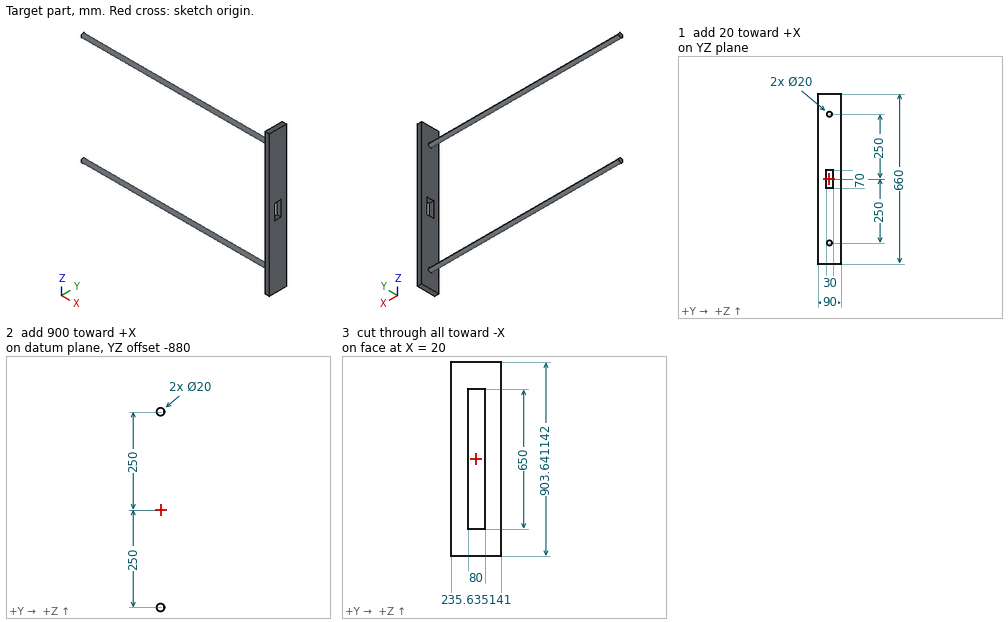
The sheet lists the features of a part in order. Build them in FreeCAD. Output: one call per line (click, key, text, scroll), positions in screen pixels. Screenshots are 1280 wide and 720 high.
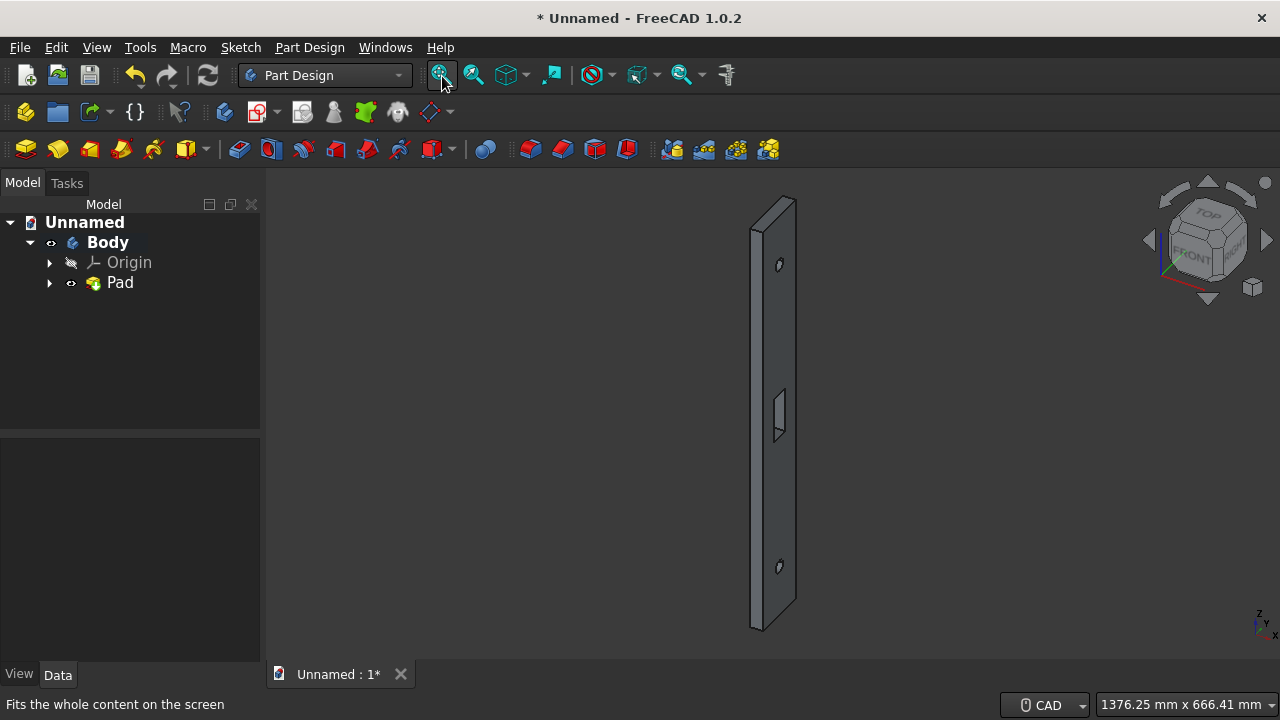
click(50, 263)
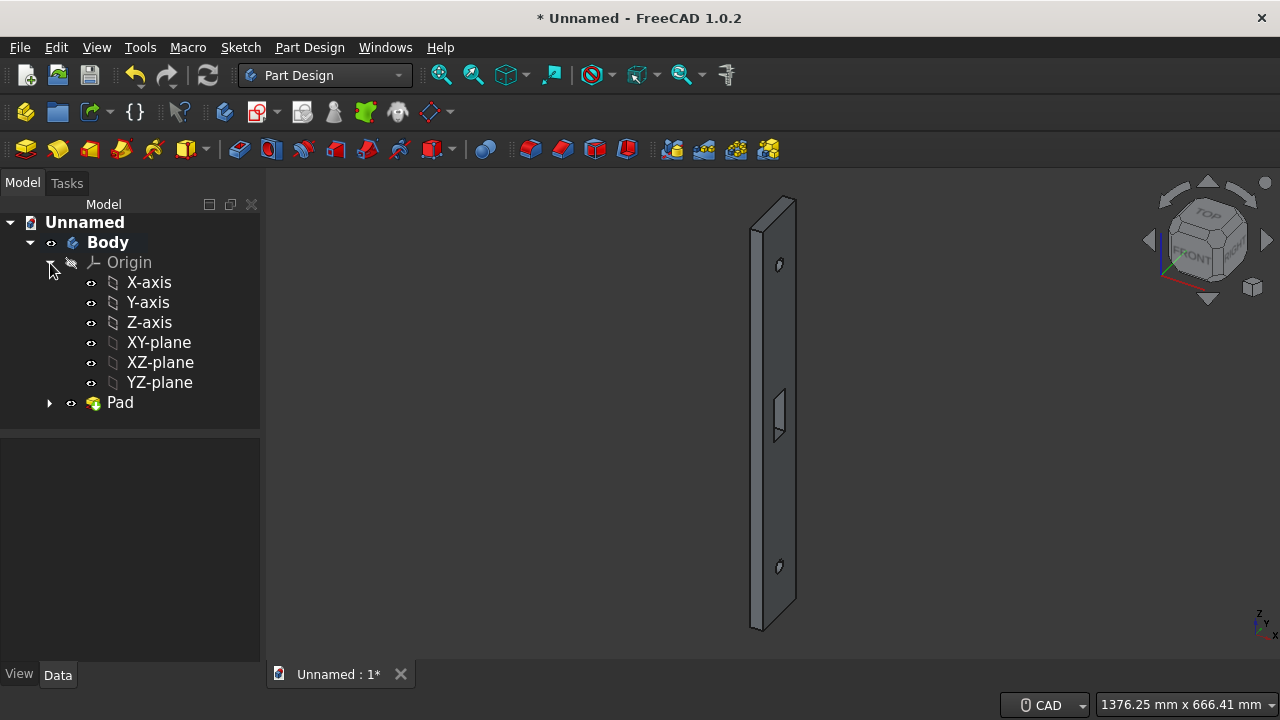
click(136, 383)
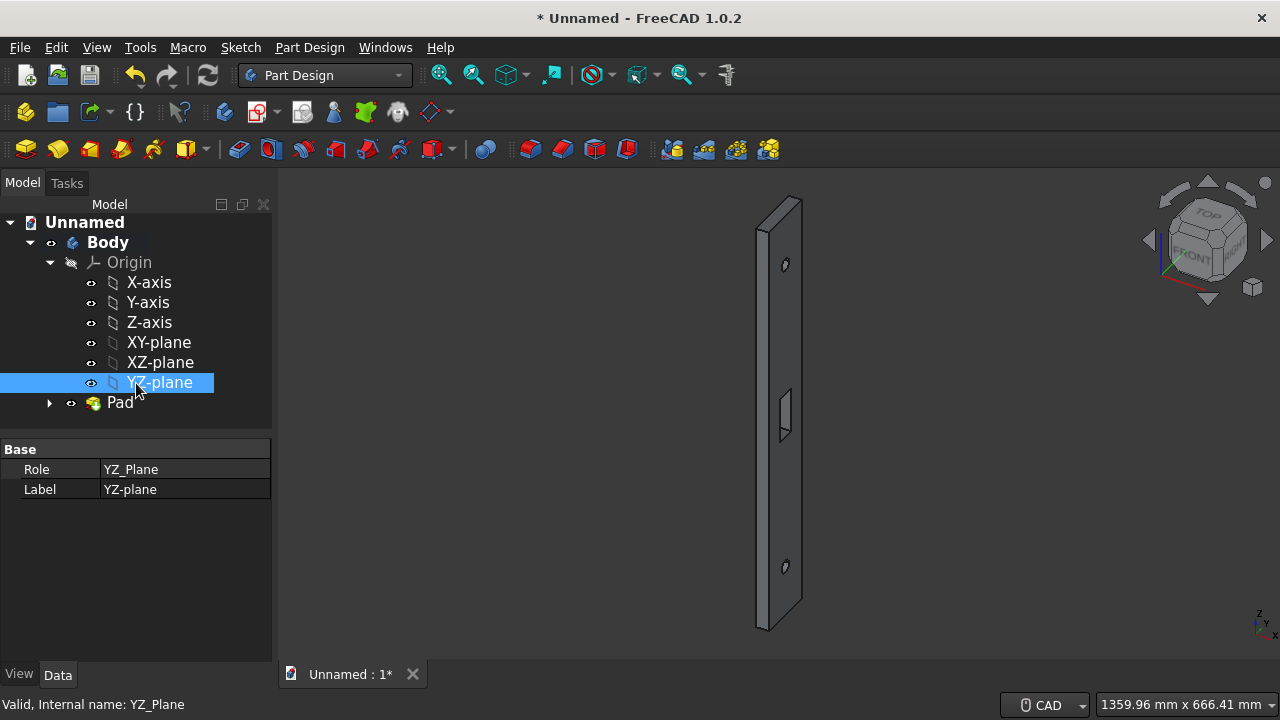
click(430, 112)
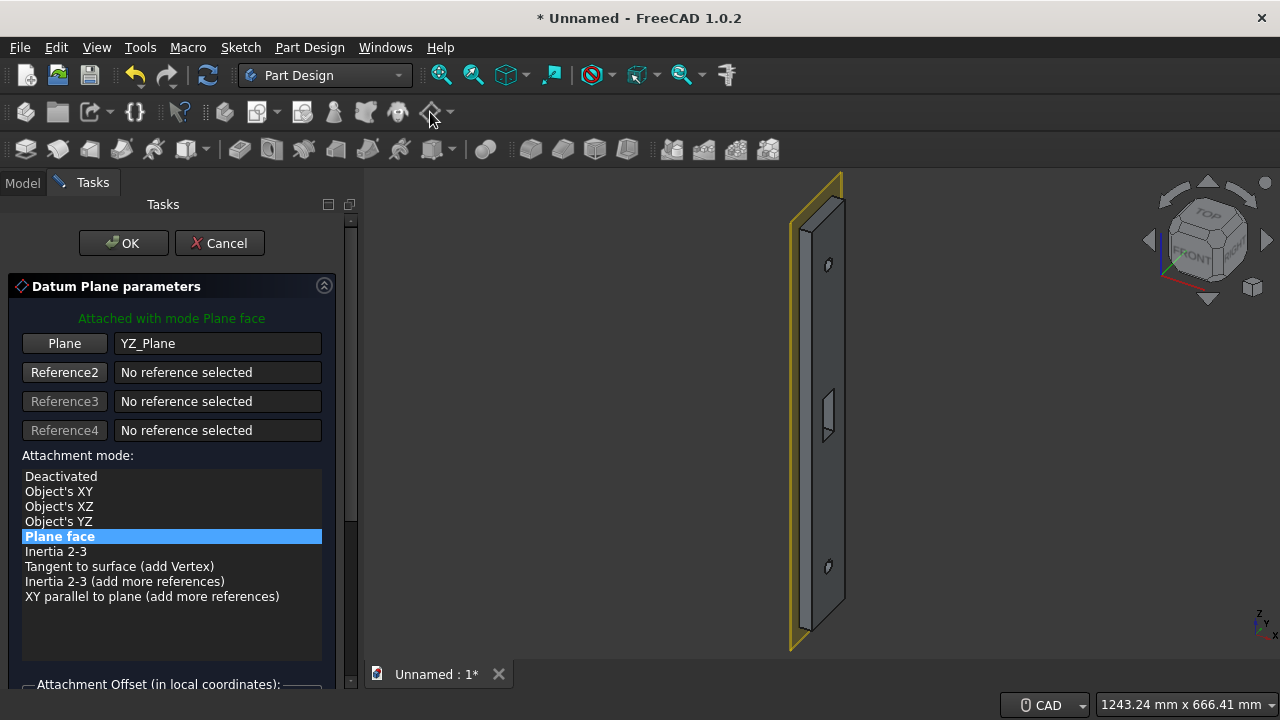
scroll(351, 451, down, 3)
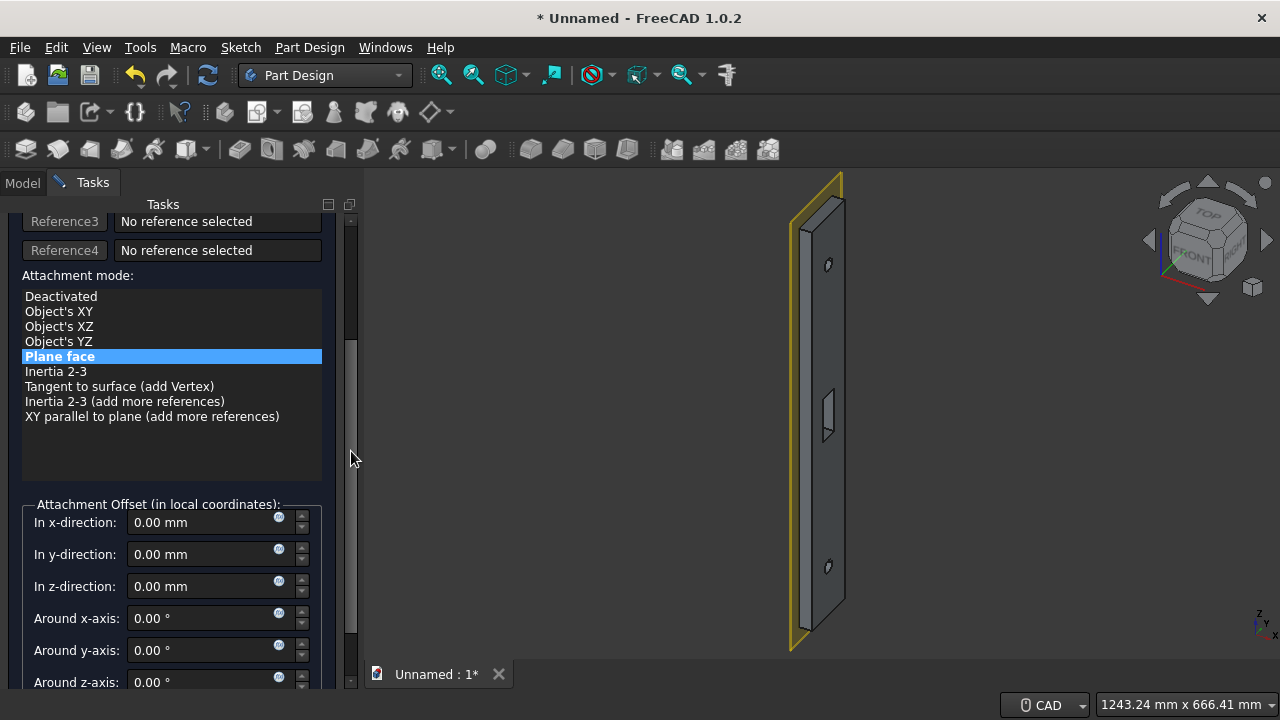
triple_click(210, 586)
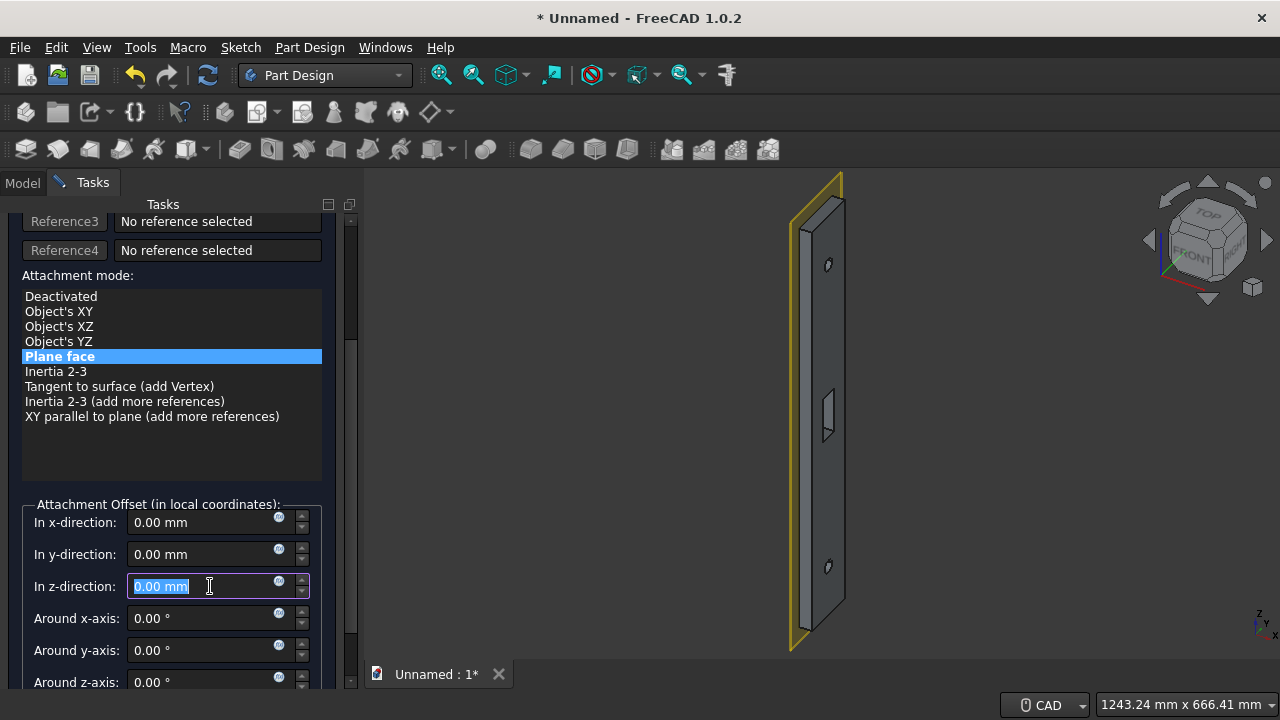
text(-880)
key(Tab)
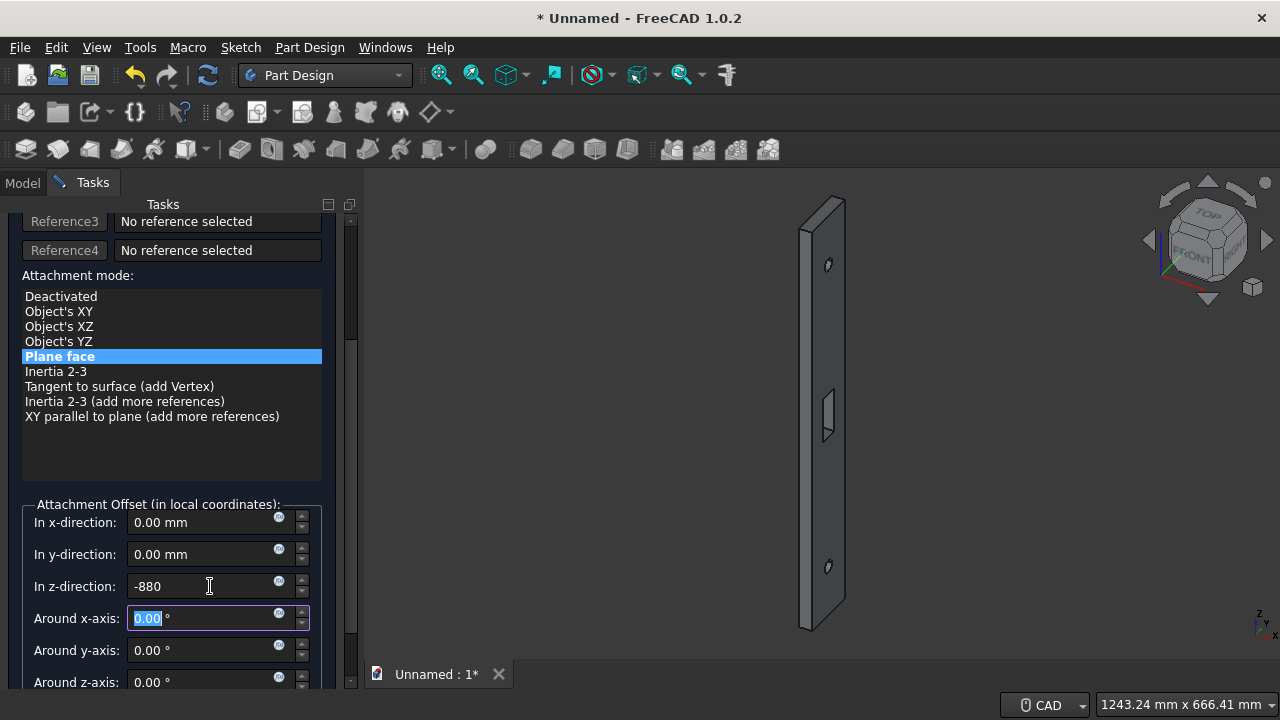
scroll(351, 451, up, 4)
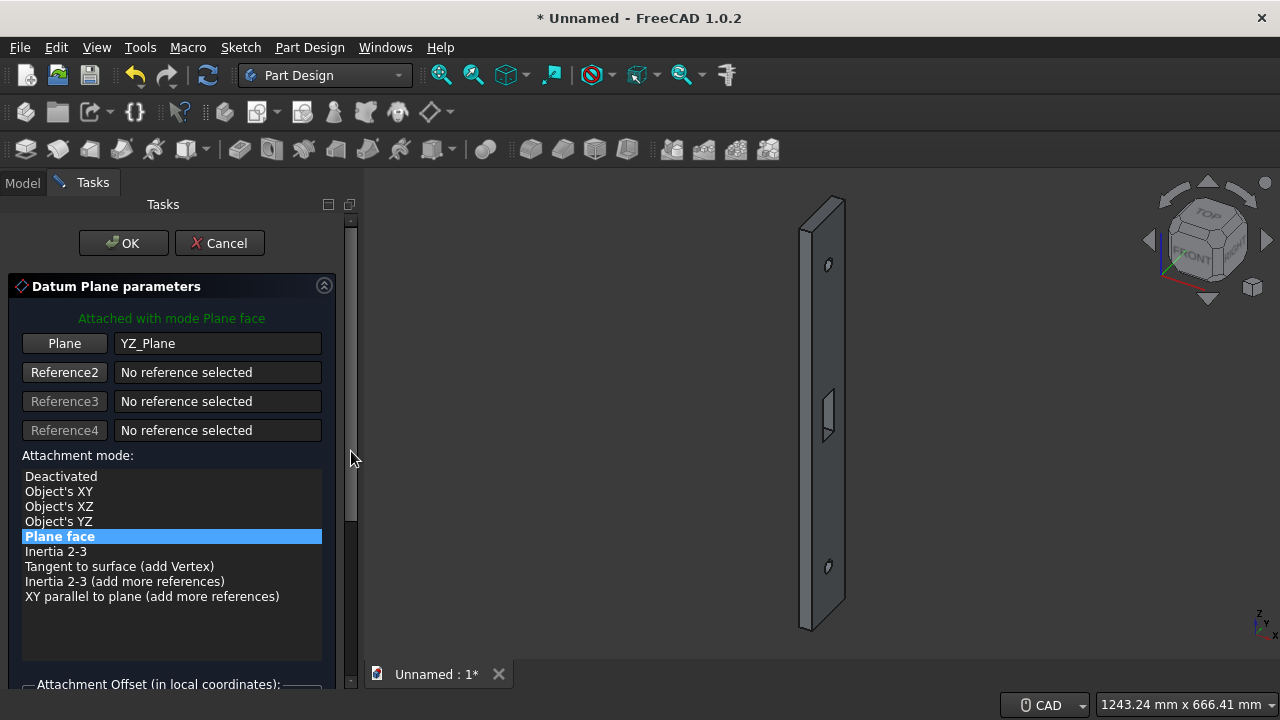
click(124, 243)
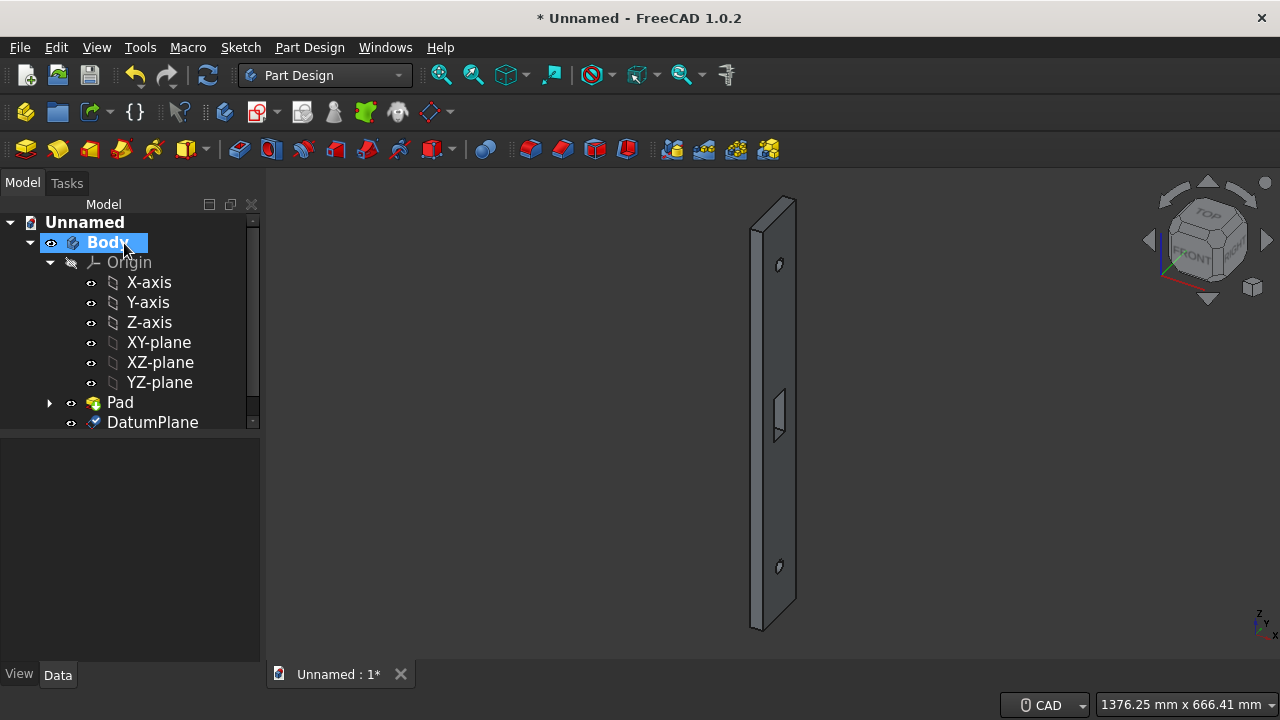
click(116, 423)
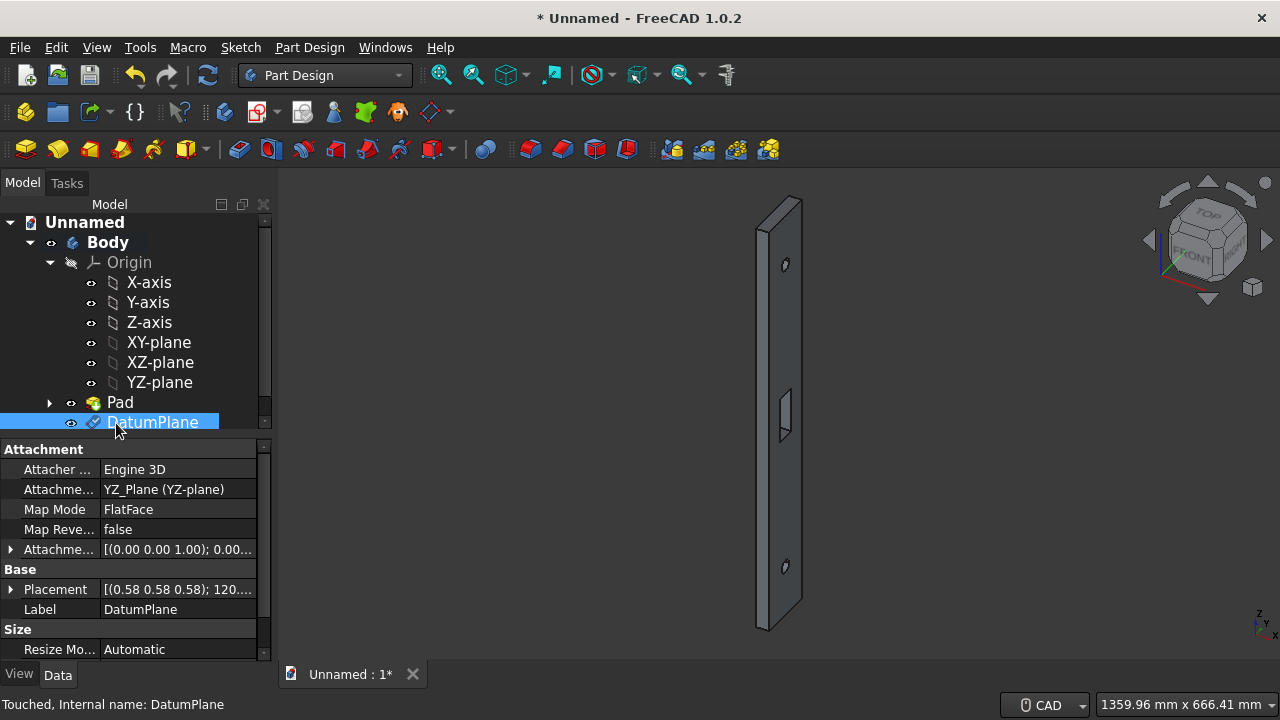
click(258, 112)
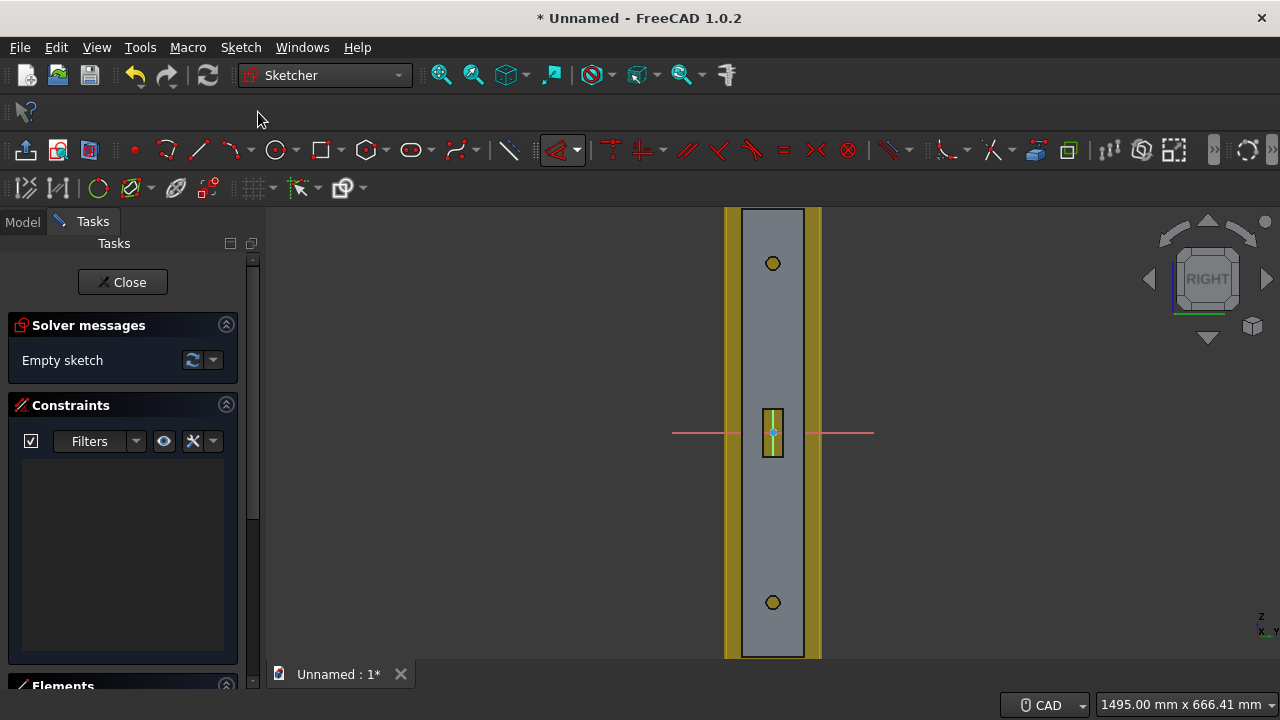
click(90, 150)